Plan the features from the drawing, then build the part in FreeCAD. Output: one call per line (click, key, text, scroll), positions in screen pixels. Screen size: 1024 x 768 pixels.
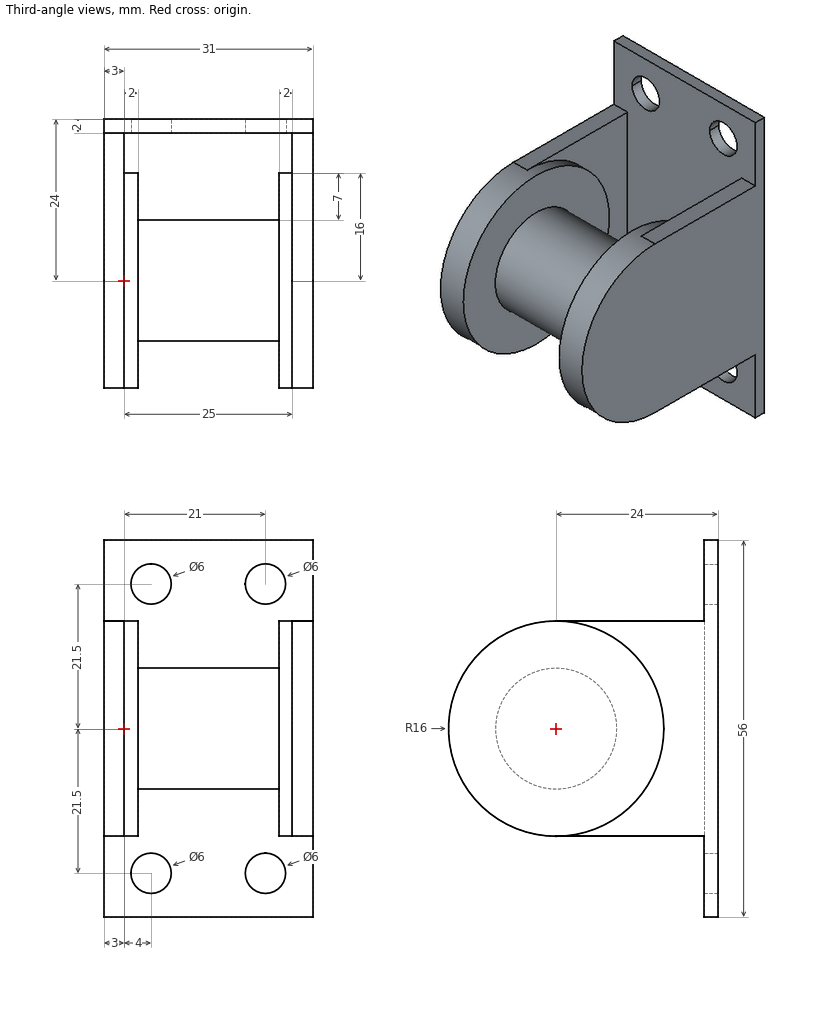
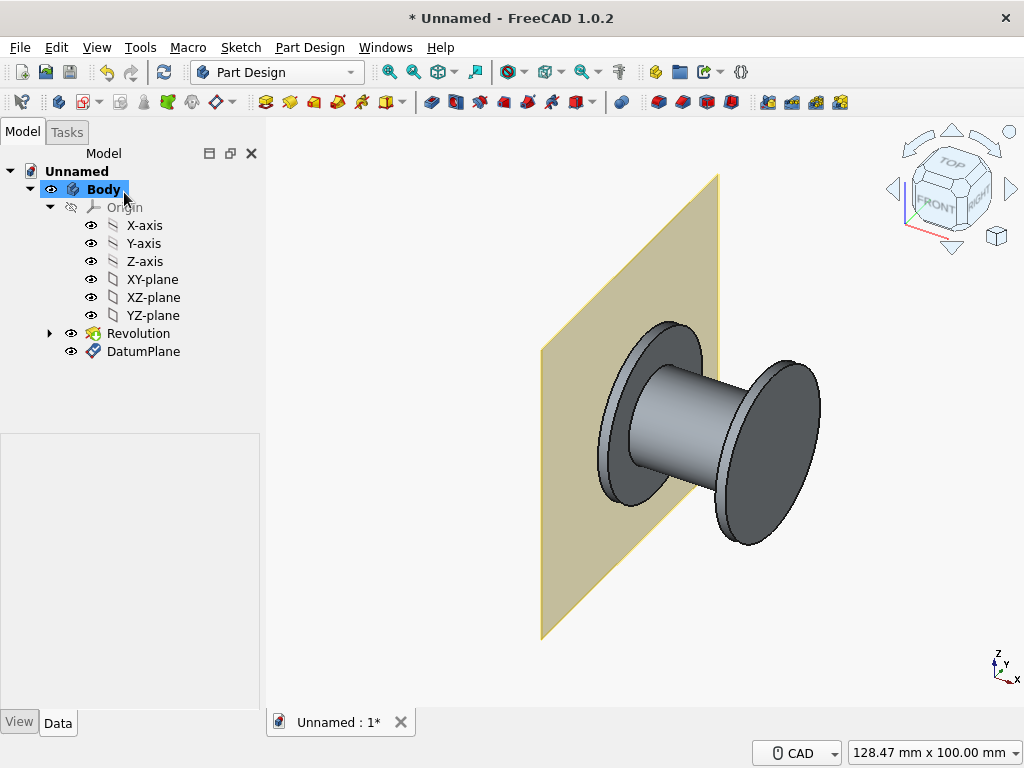
click(116, 351)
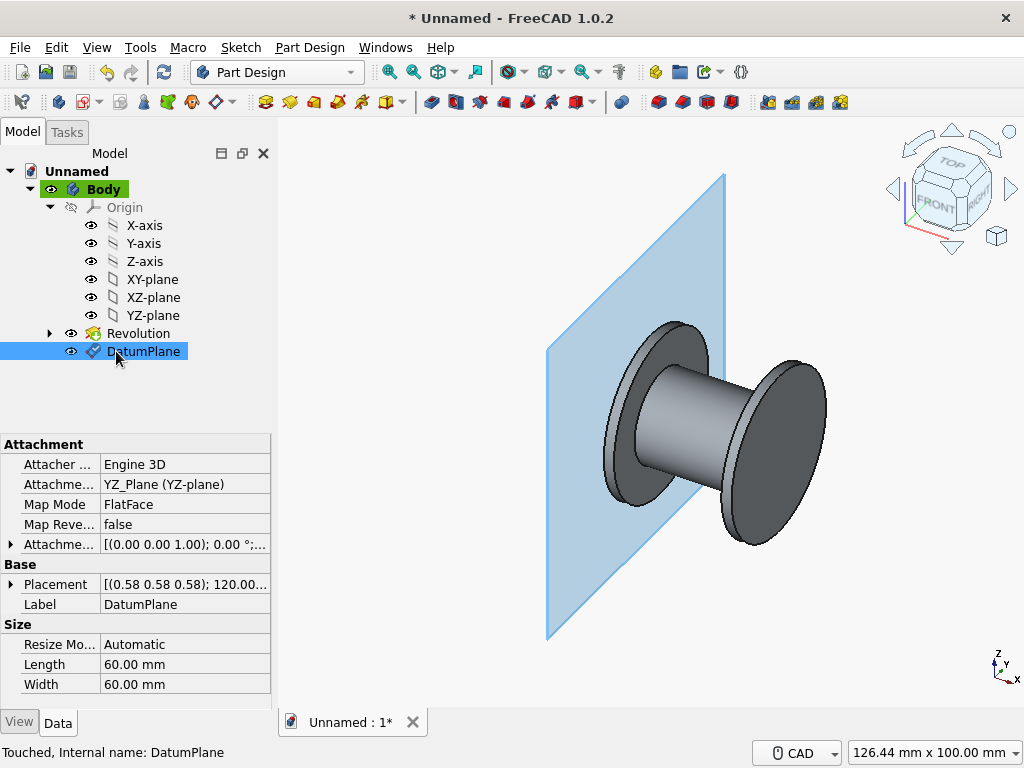
click(84, 102)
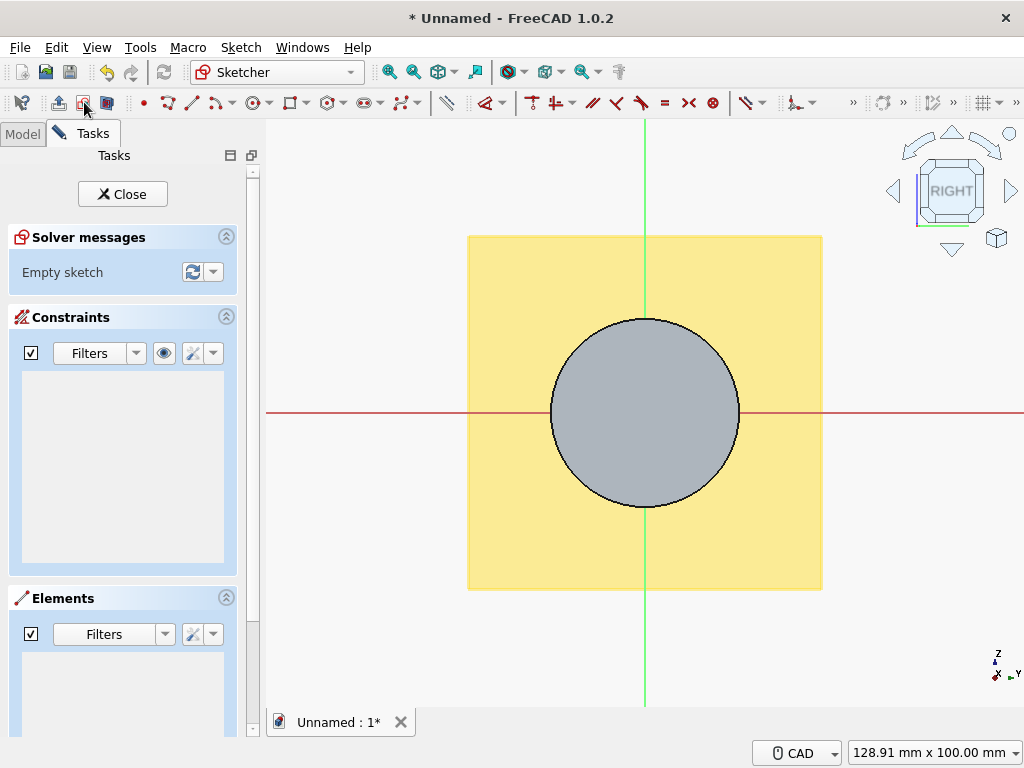
click(108, 104)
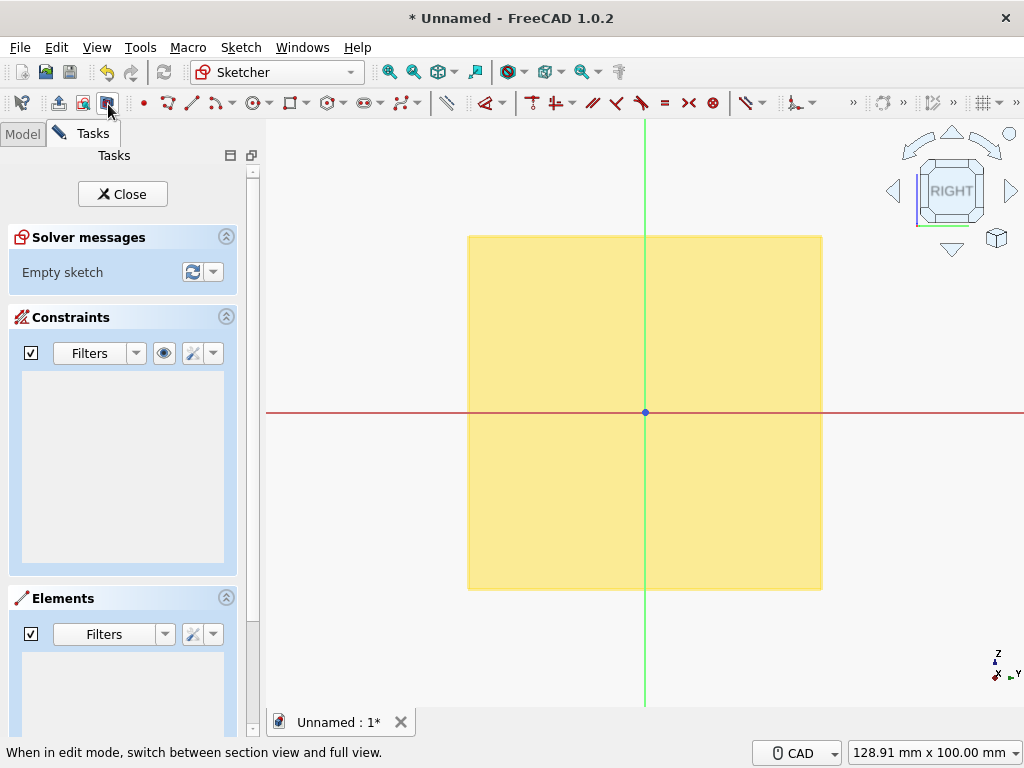
scroll(780, 413, up, 3)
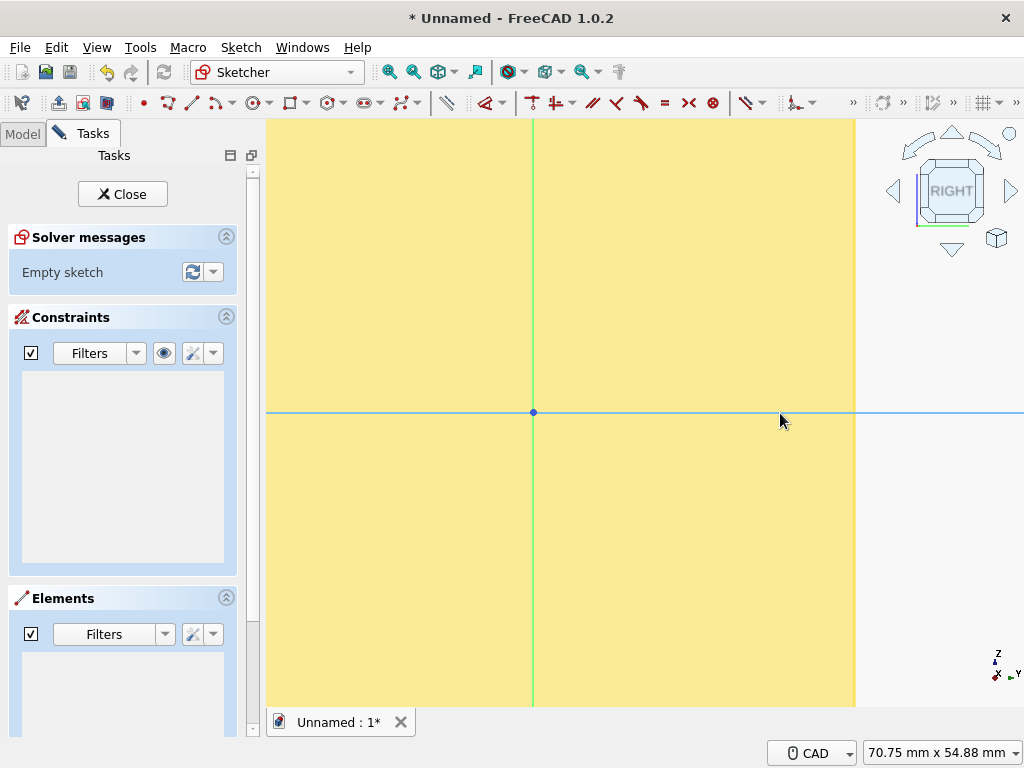
click(168, 104)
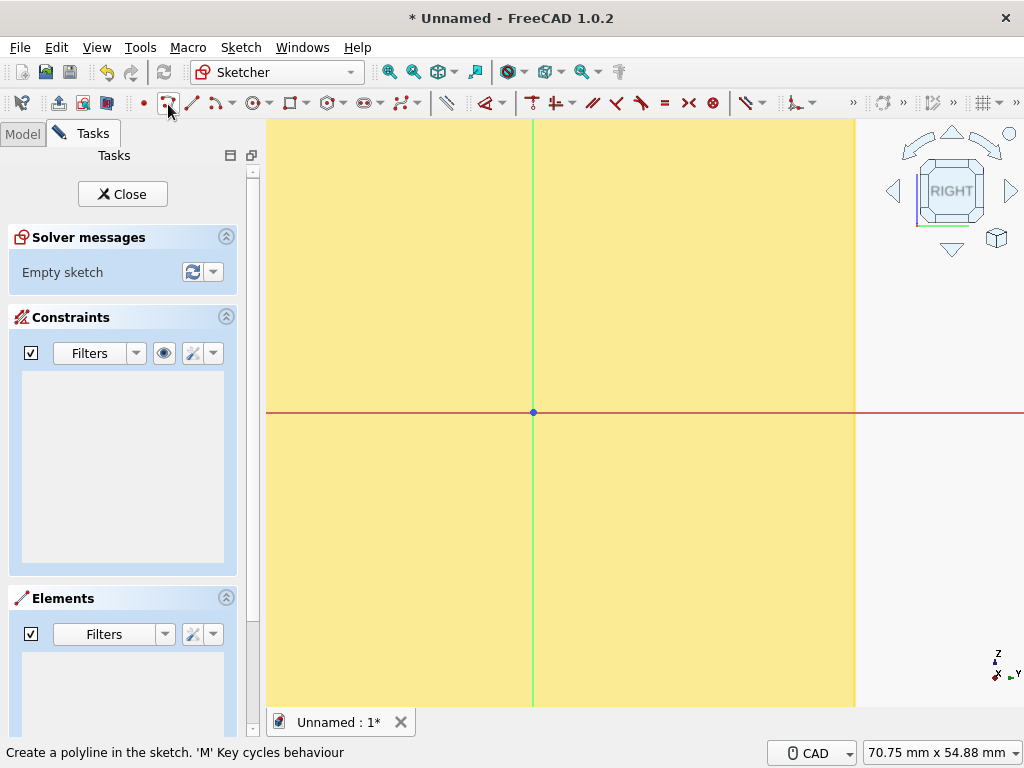
click(533, 241)
click(791, 241)
click(791, 584)
click(533, 584)
right_click(533, 584)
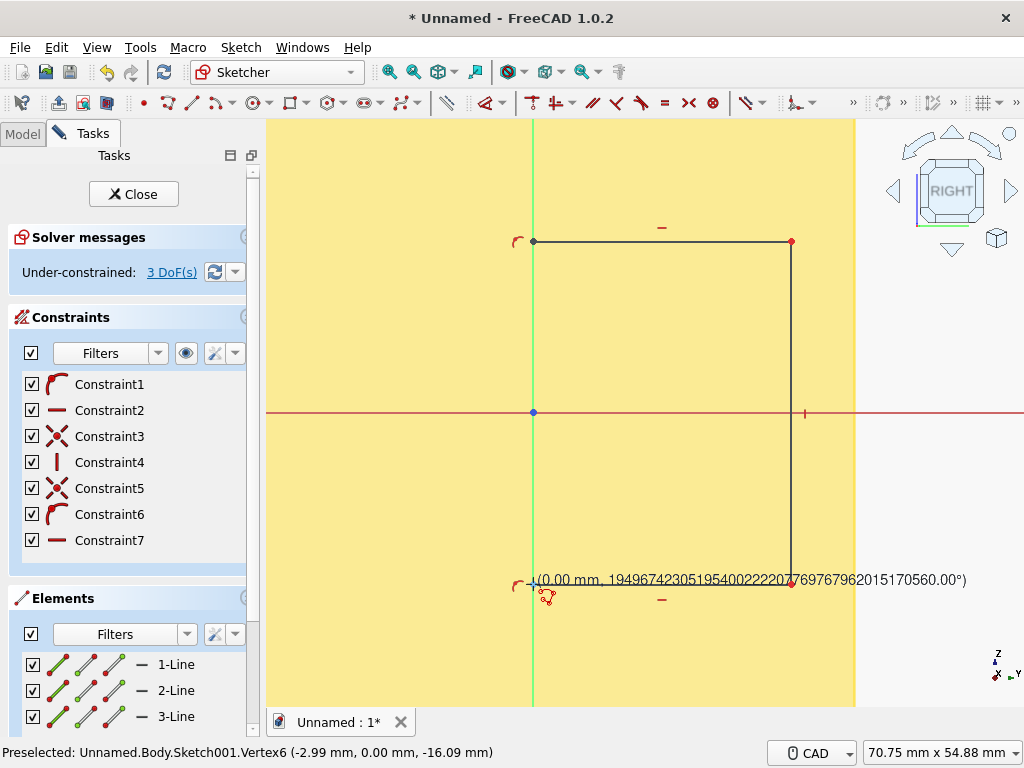
click(234, 104)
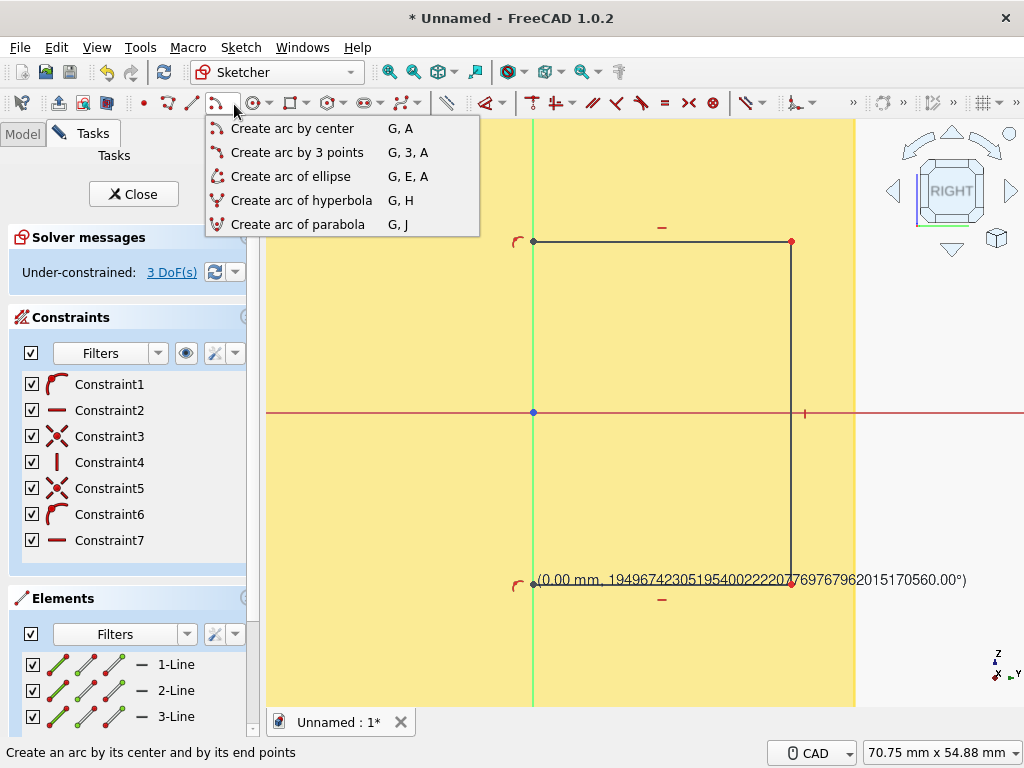
click(342, 152)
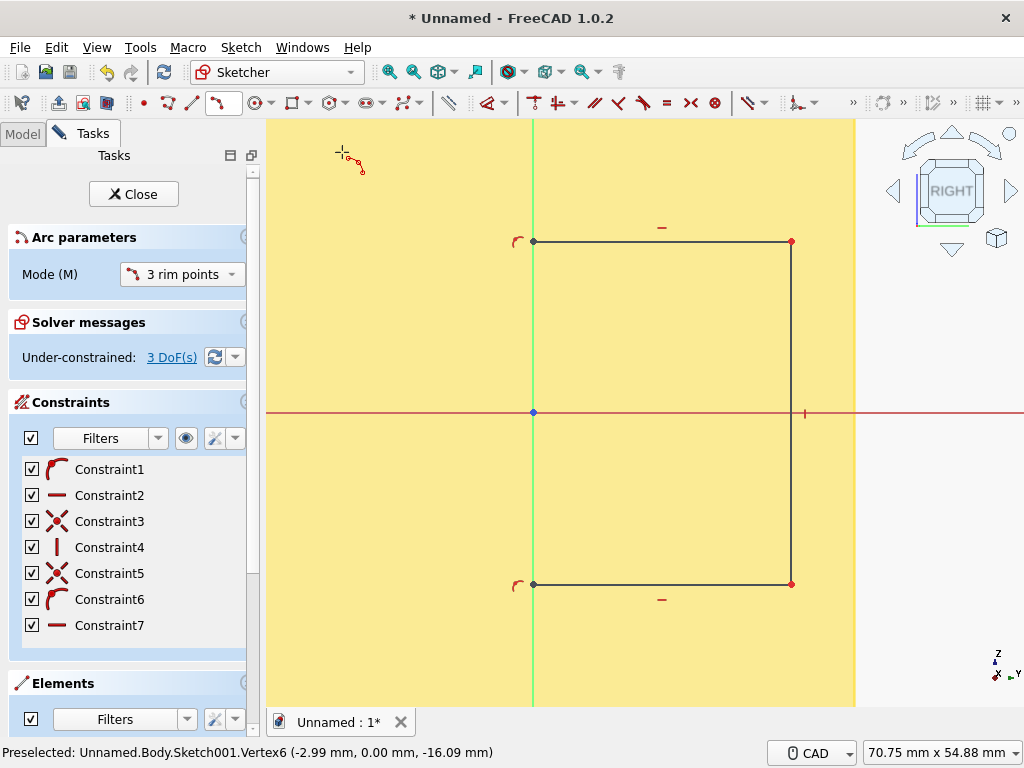
click(533, 585)
click(533, 242)
click(370, 360)
key(Escape)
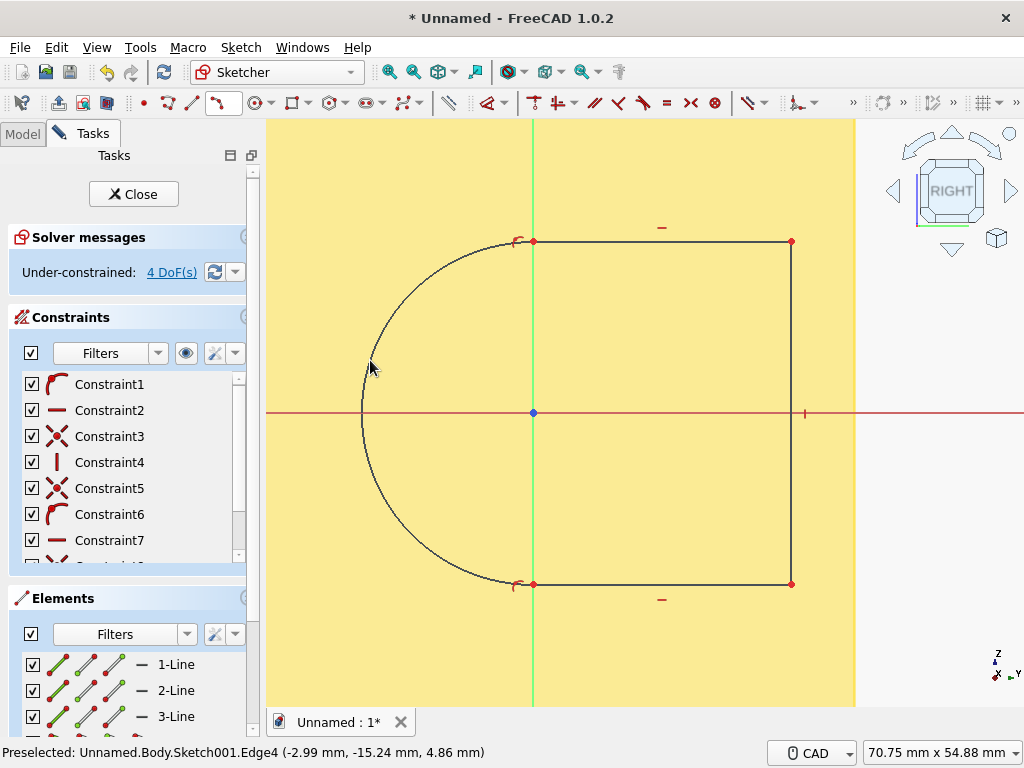
click(611, 242)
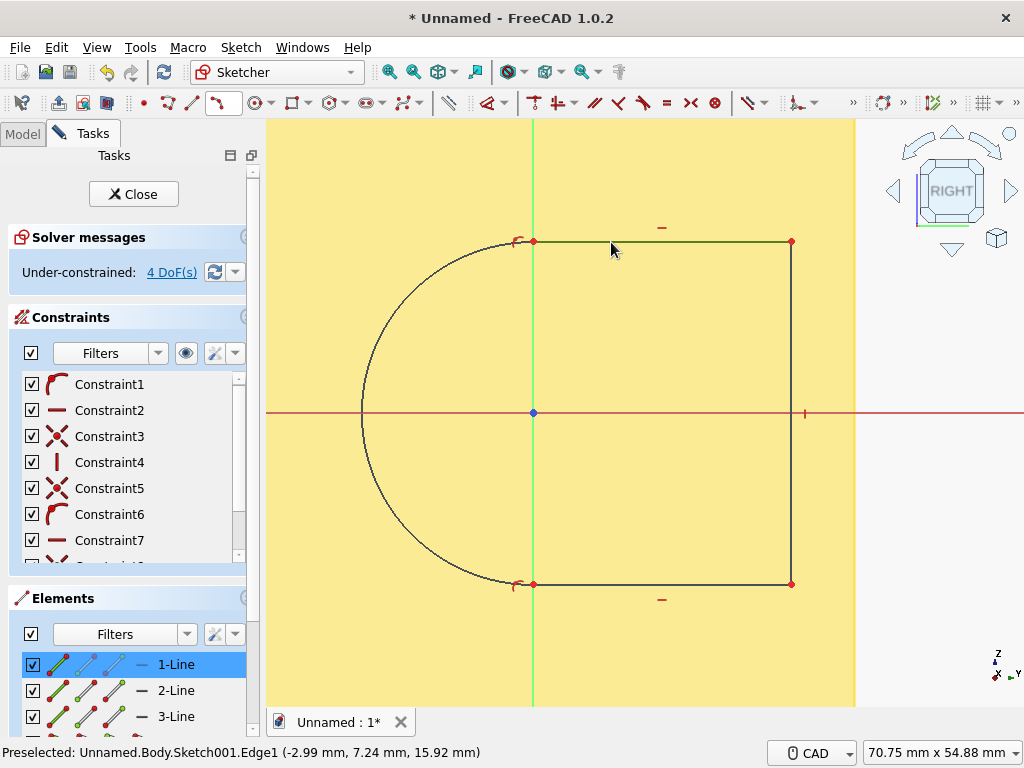
click(395, 313)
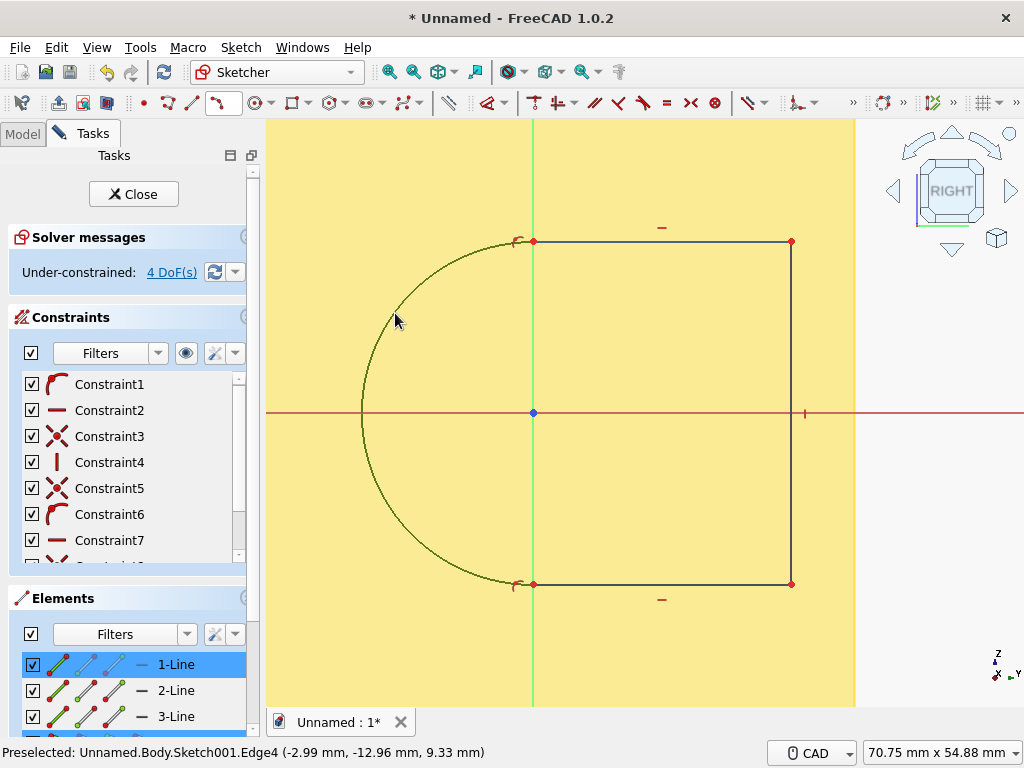
click(644, 104)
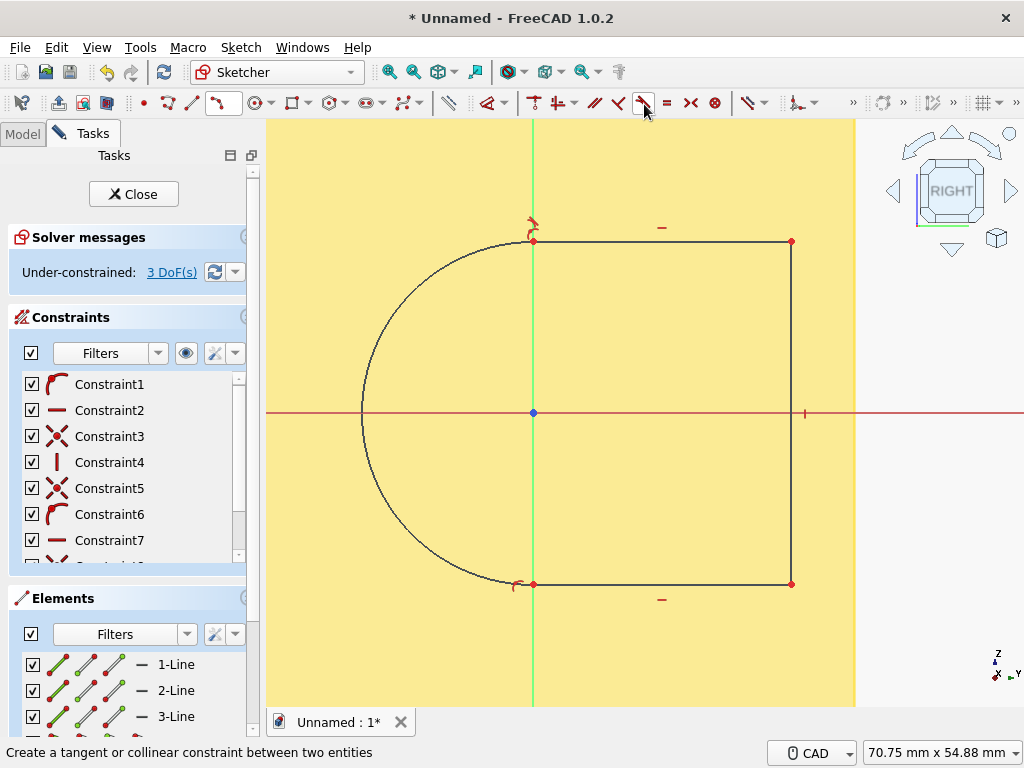
click(533, 414)